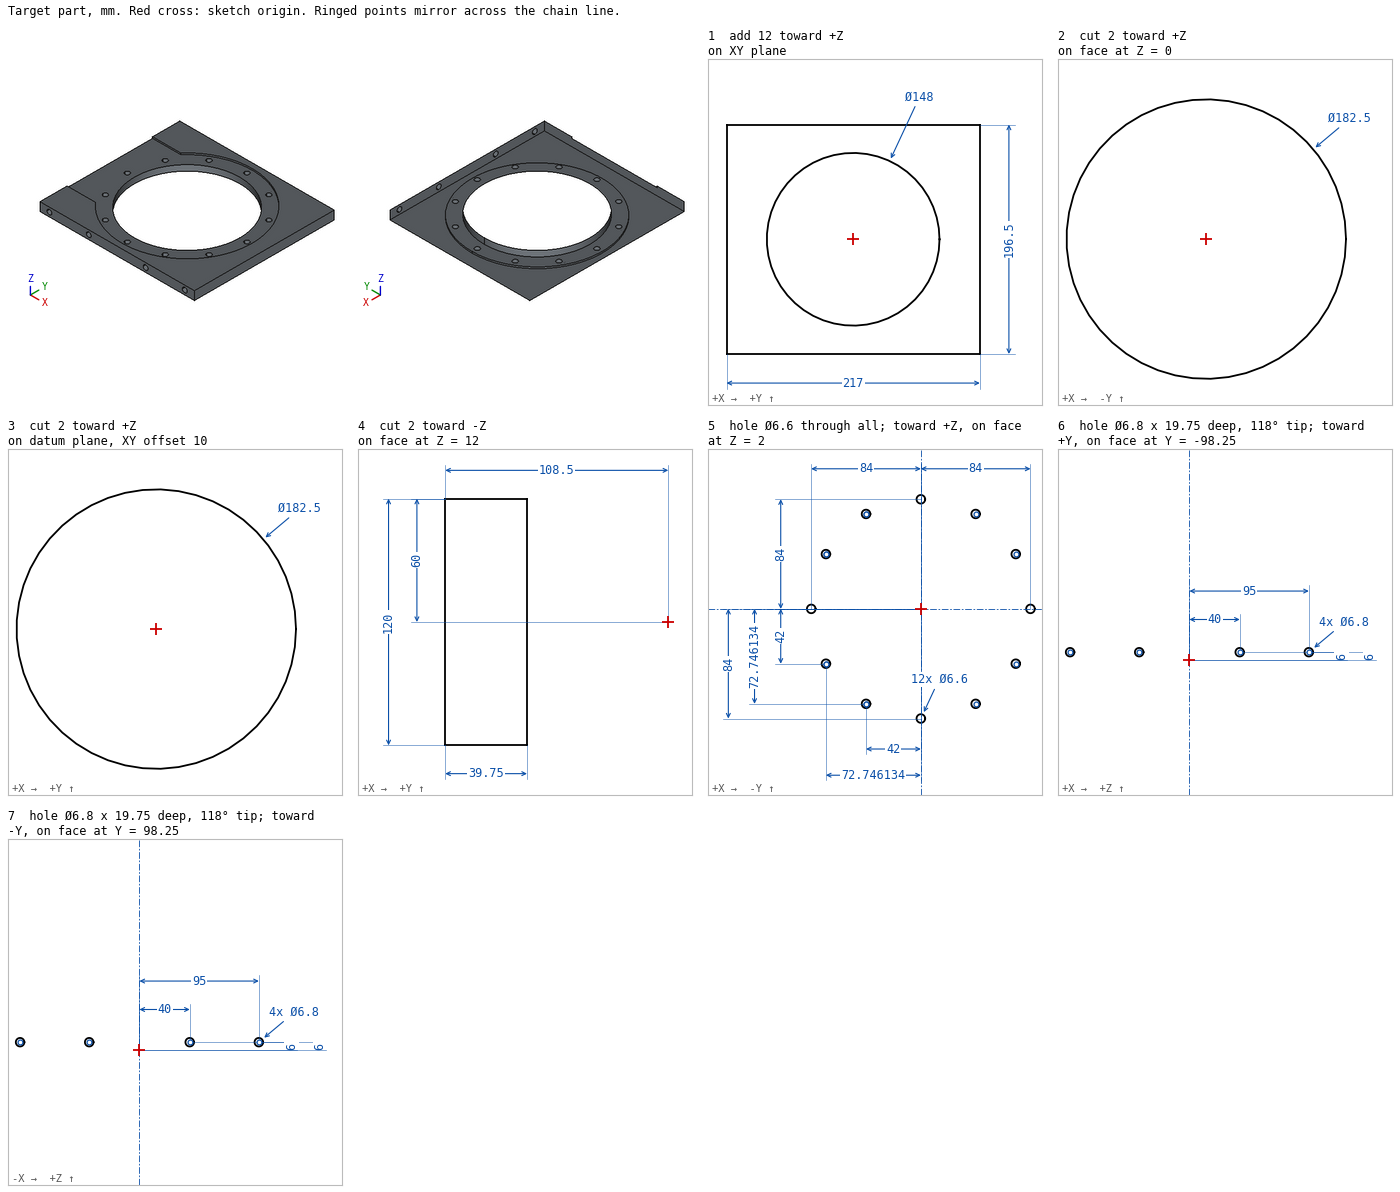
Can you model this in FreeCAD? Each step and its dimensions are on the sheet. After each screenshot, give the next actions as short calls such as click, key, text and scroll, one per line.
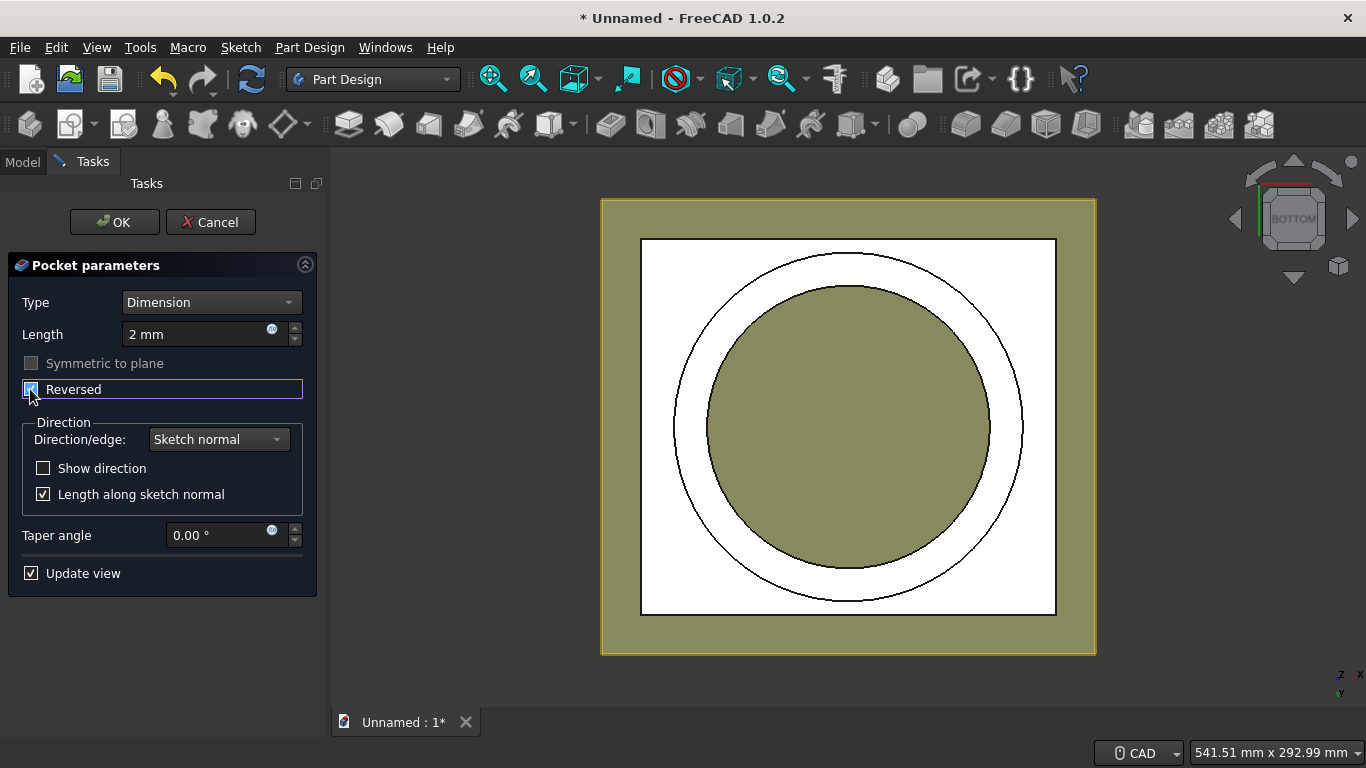
click(115, 222)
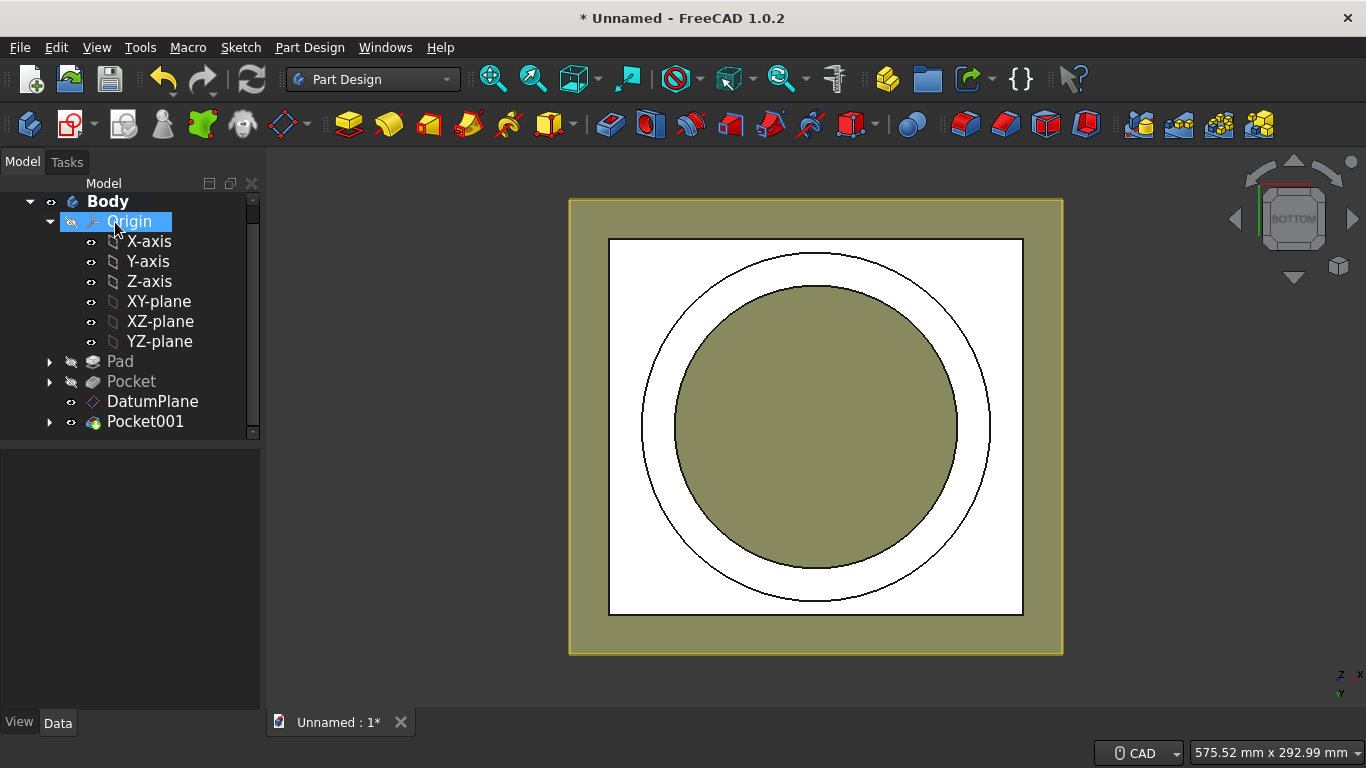
click(116, 402)
key(space)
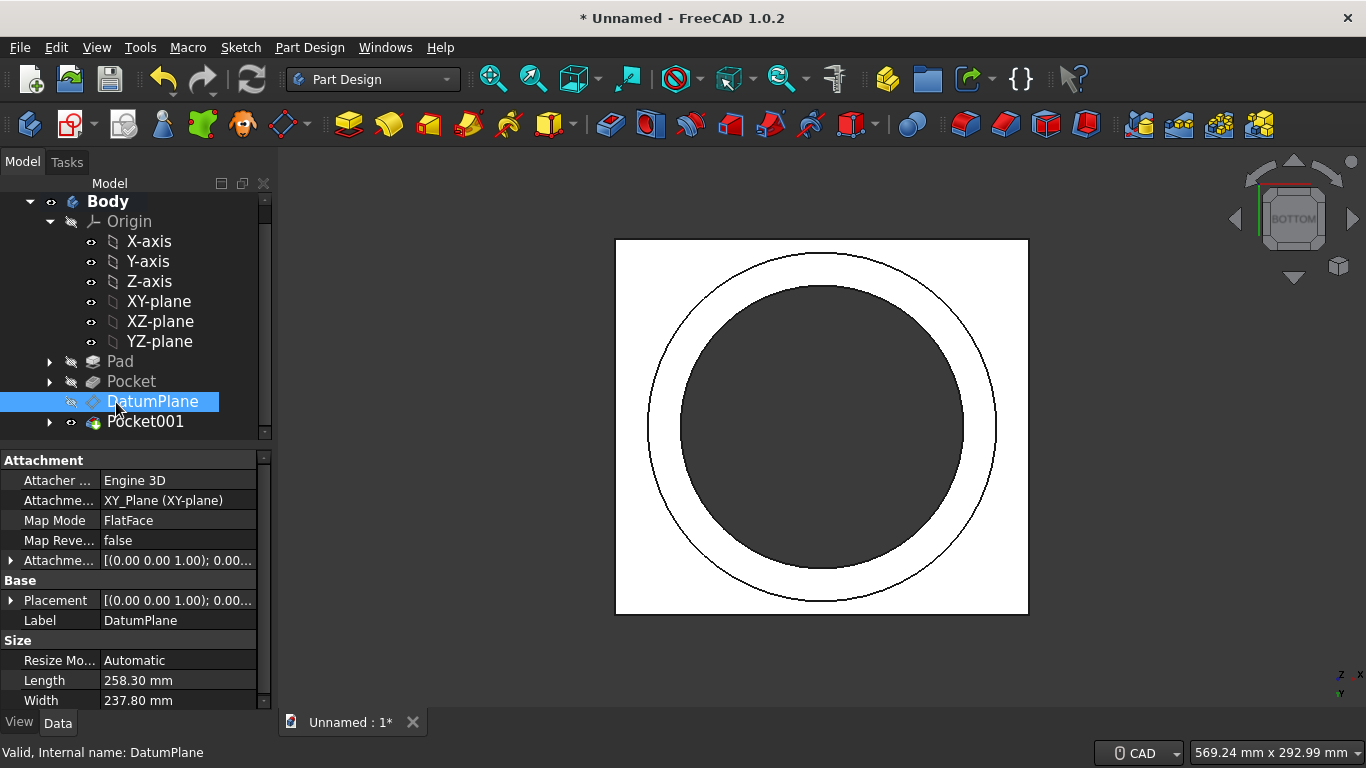
key(0)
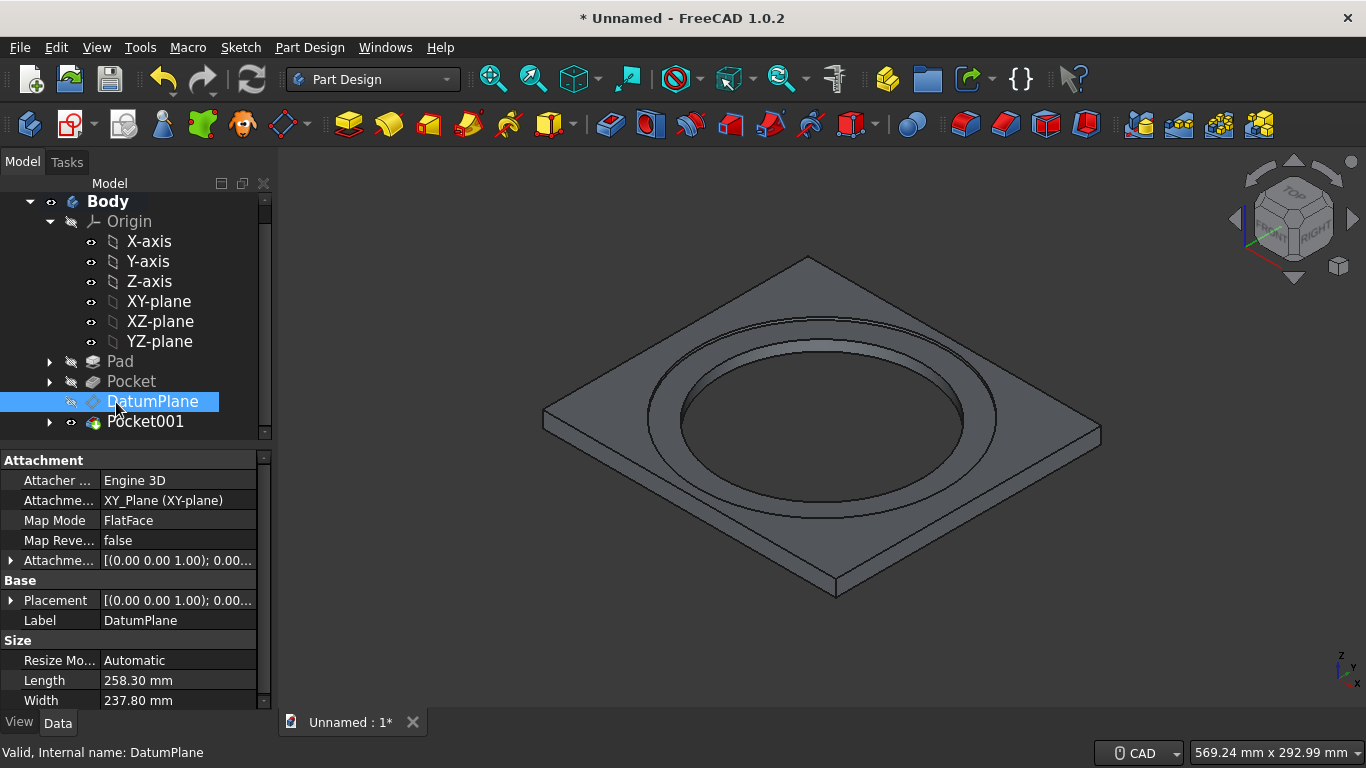
click(1024, 445)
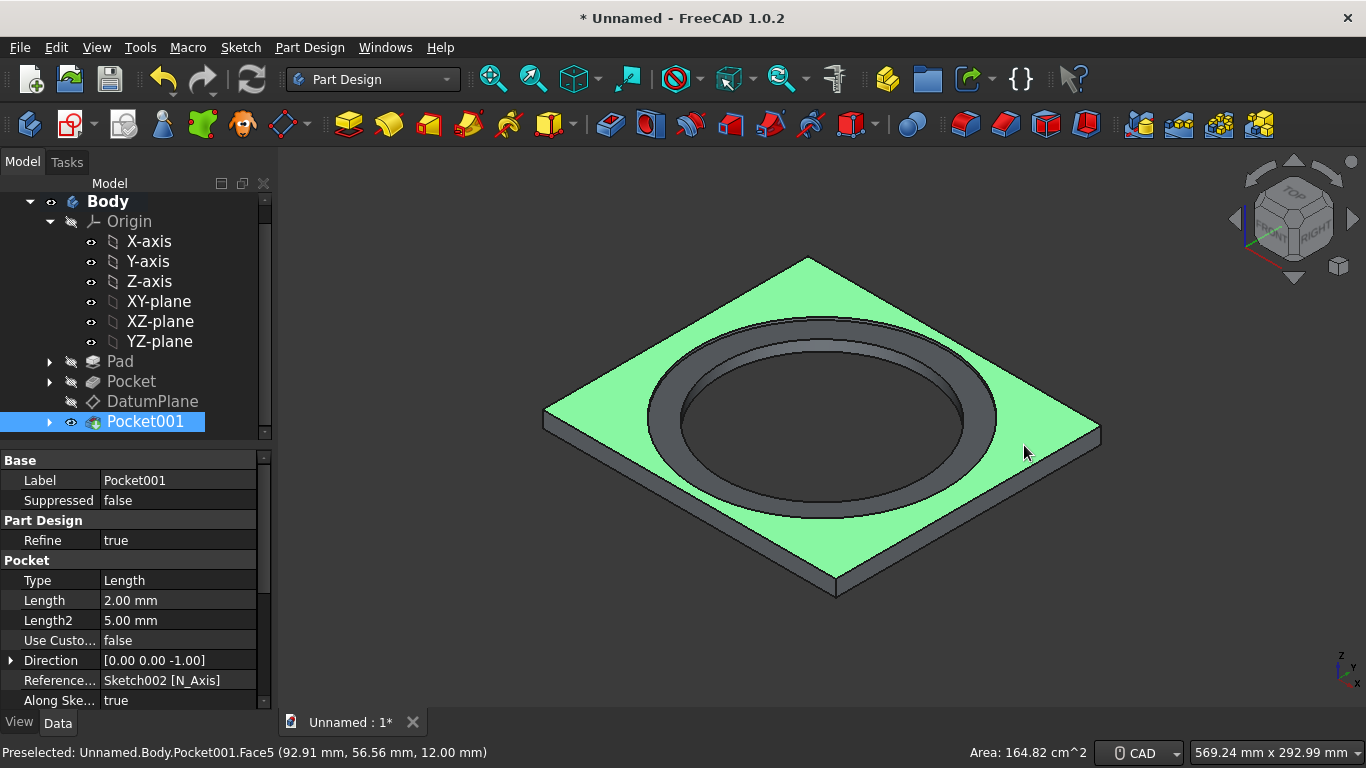
click(70, 124)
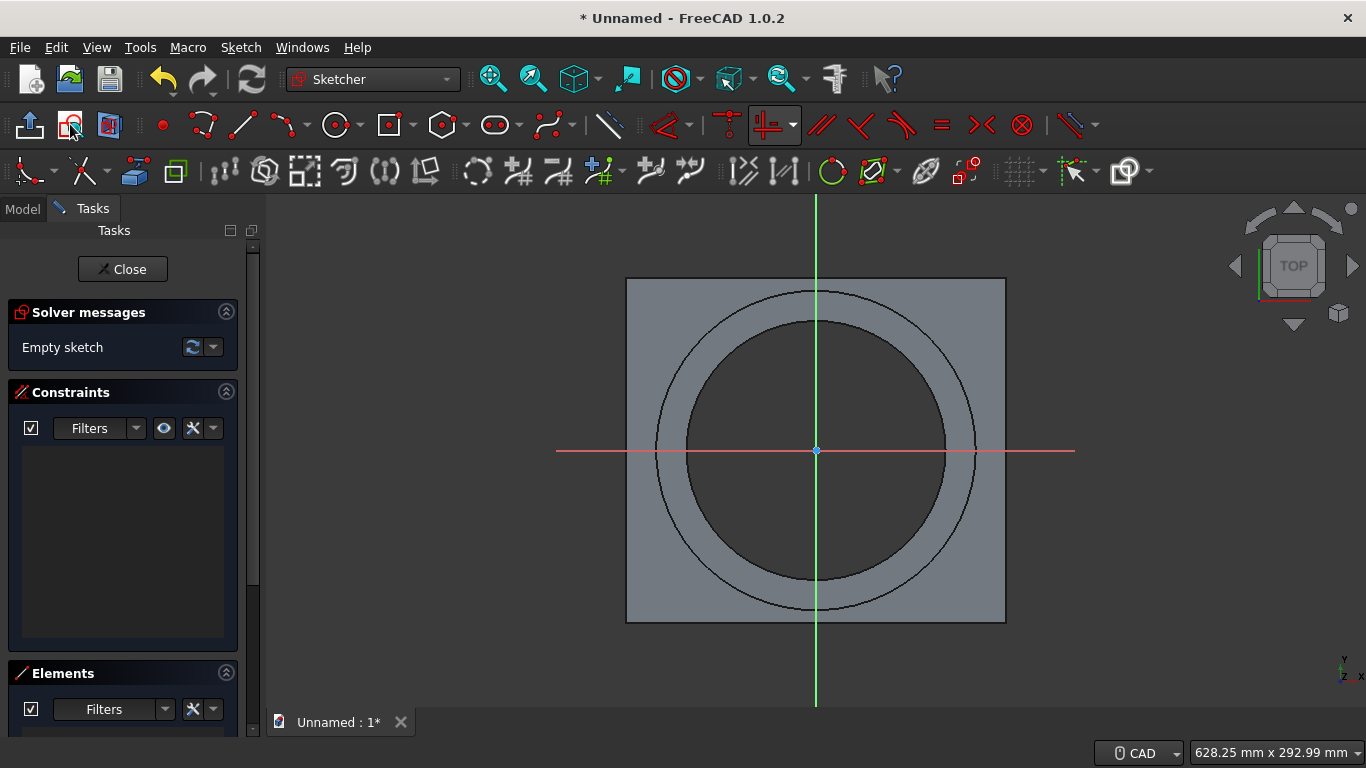
scroll(667, 450, up, 2)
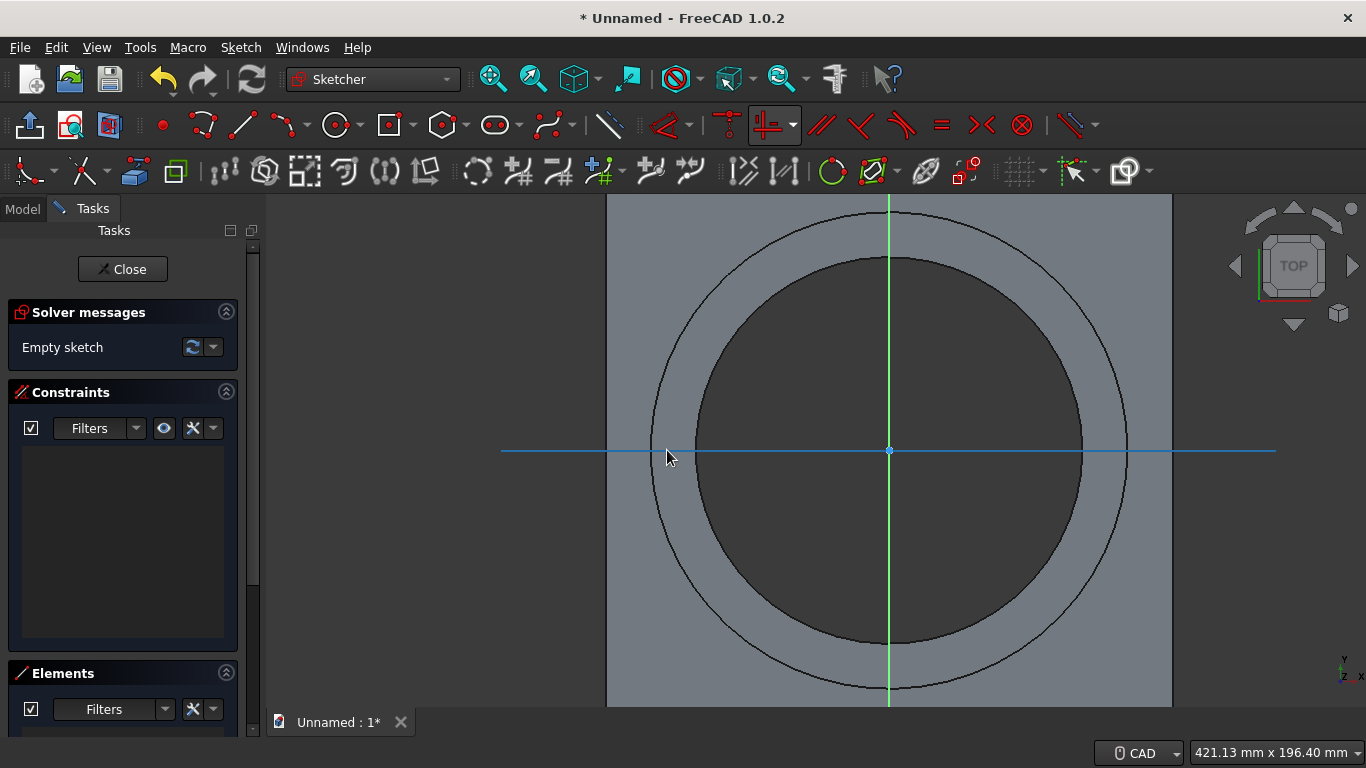
click(416, 126)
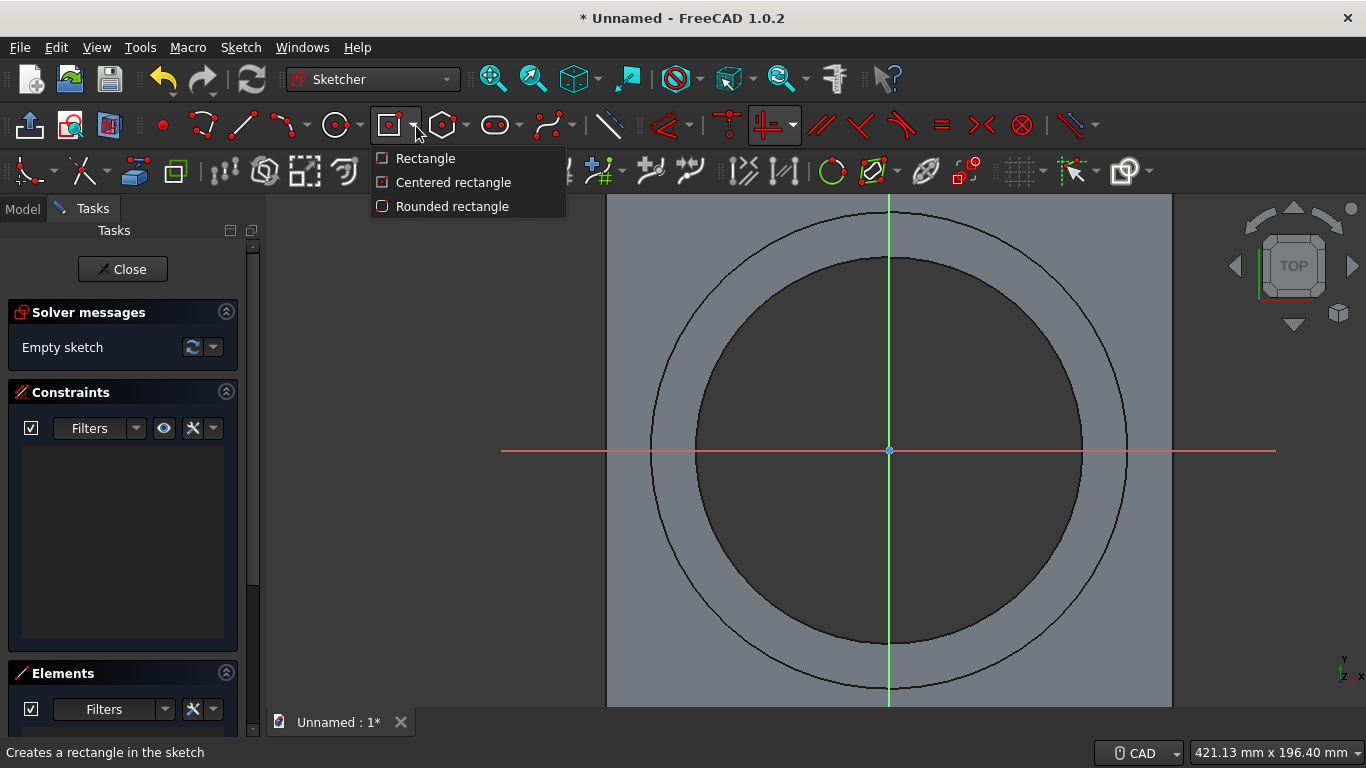
click(468, 158)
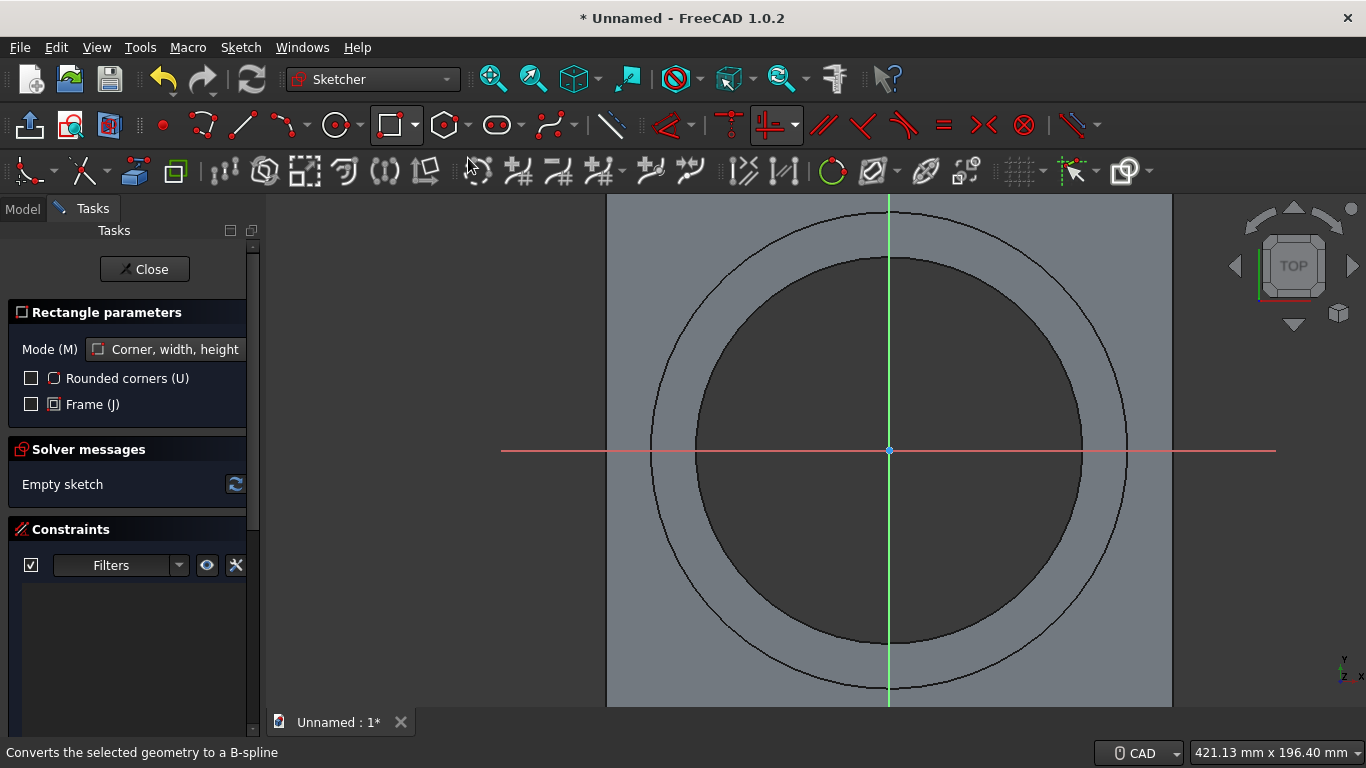
click(606, 294)
click(710, 607)
key(Escape)